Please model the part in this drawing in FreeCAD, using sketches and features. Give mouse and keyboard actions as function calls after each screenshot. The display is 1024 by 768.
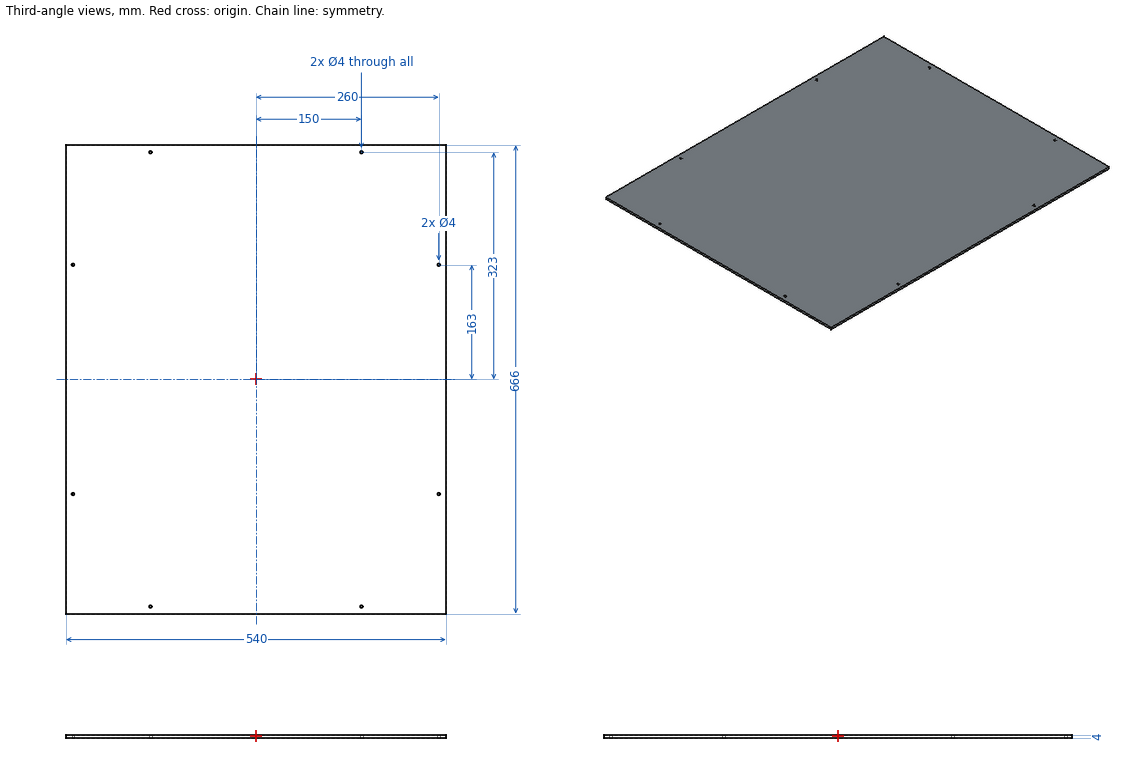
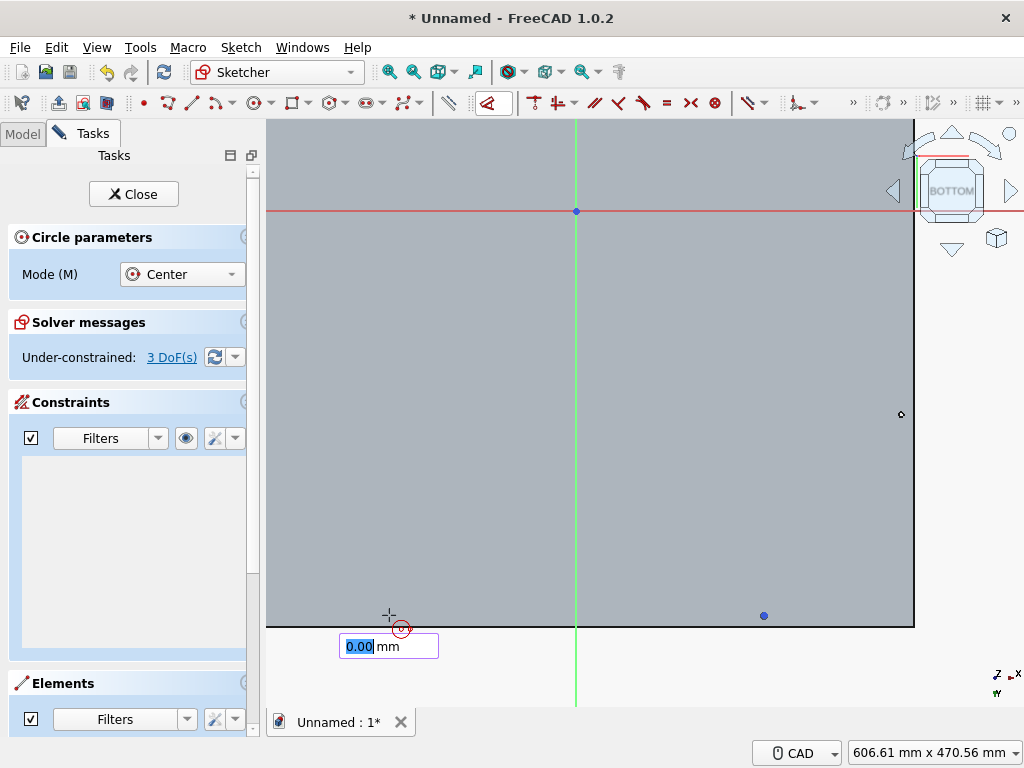
scroll(391, 613, up, 10)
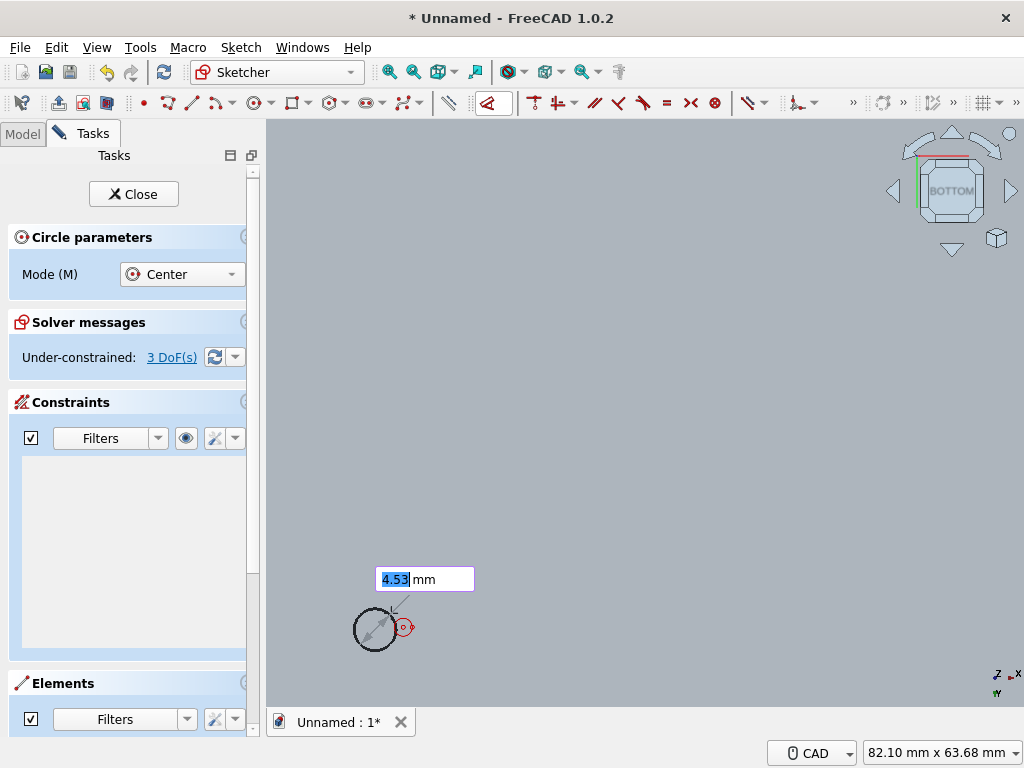
click(387, 606)
key(Escape)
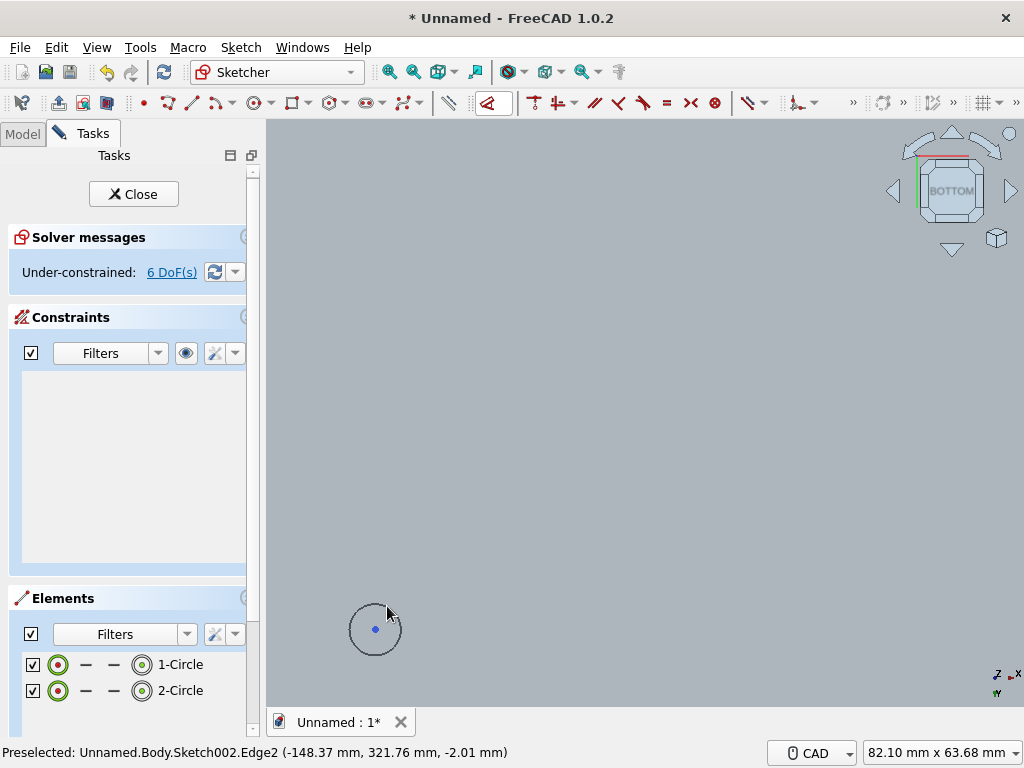
scroll(391, 613, down, 10)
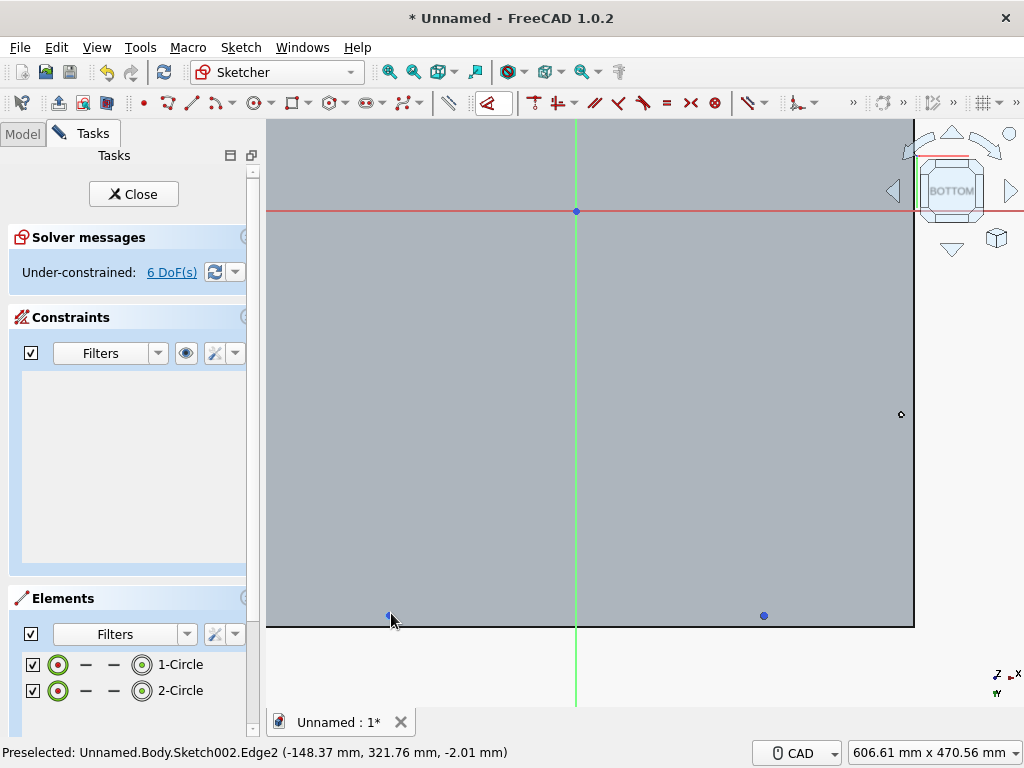
scroll(766, 614, up, 8)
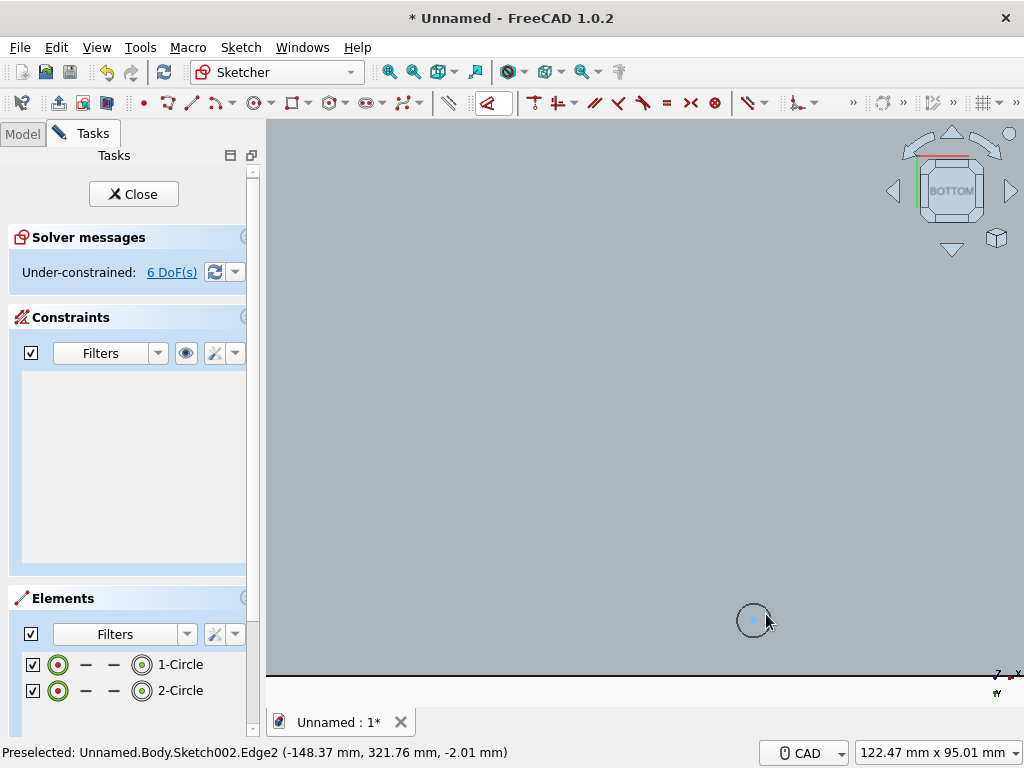
click(766, 609)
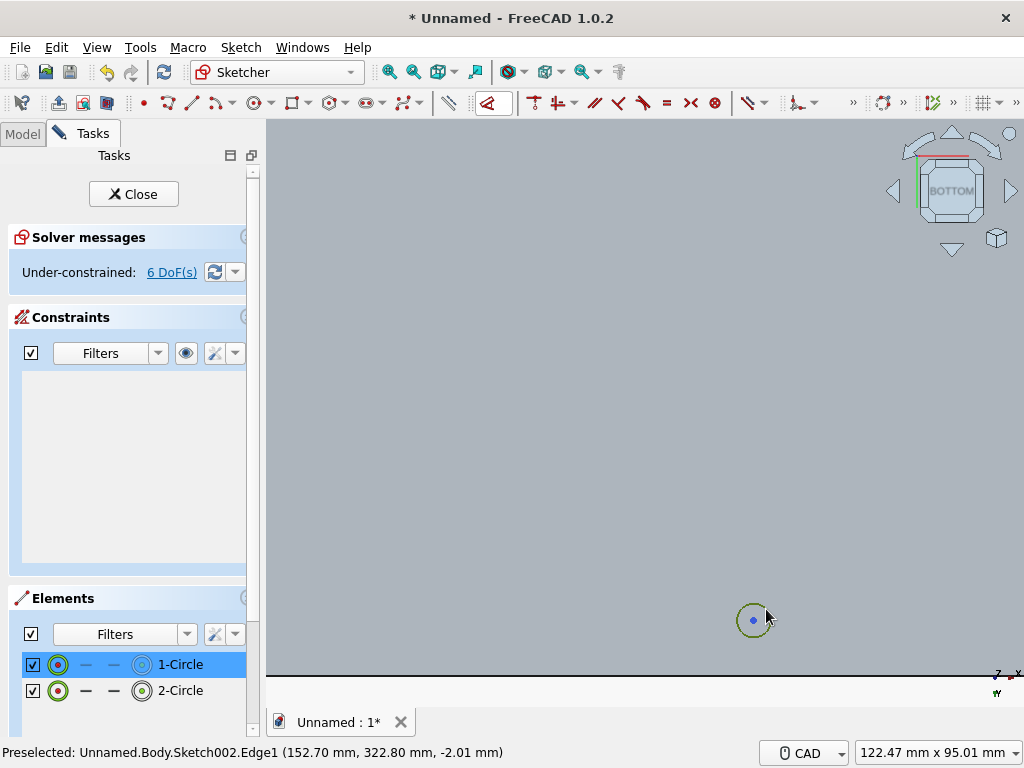
scroll(767, 614, down, 8)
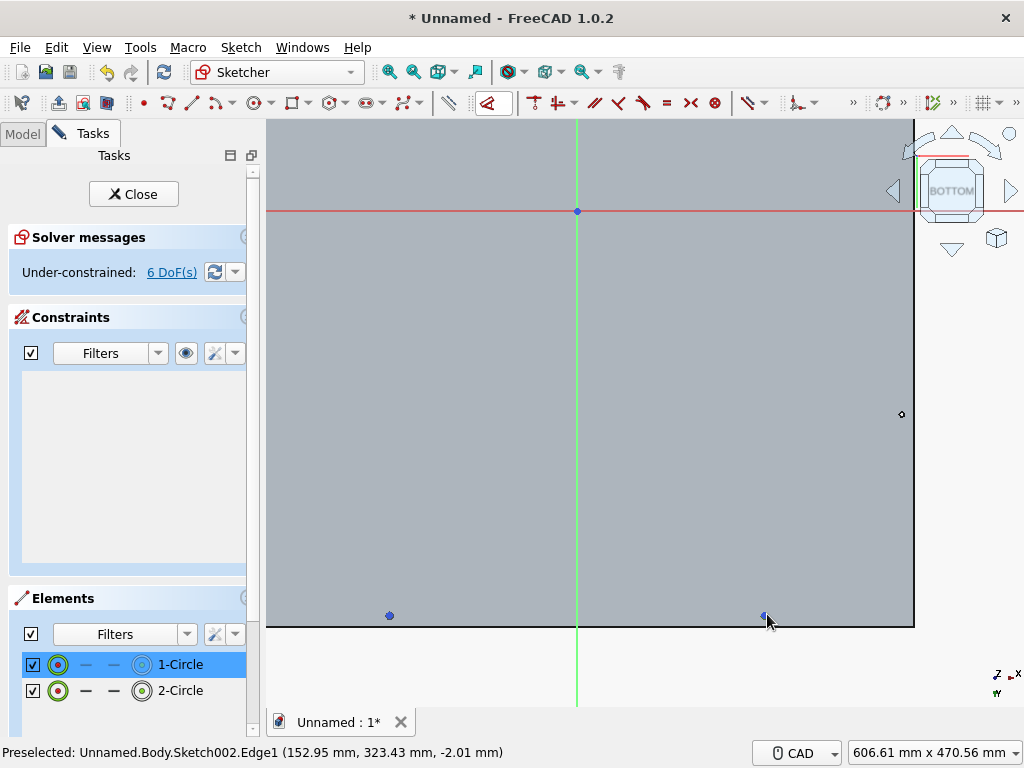
scroll(392, 614, up, 7)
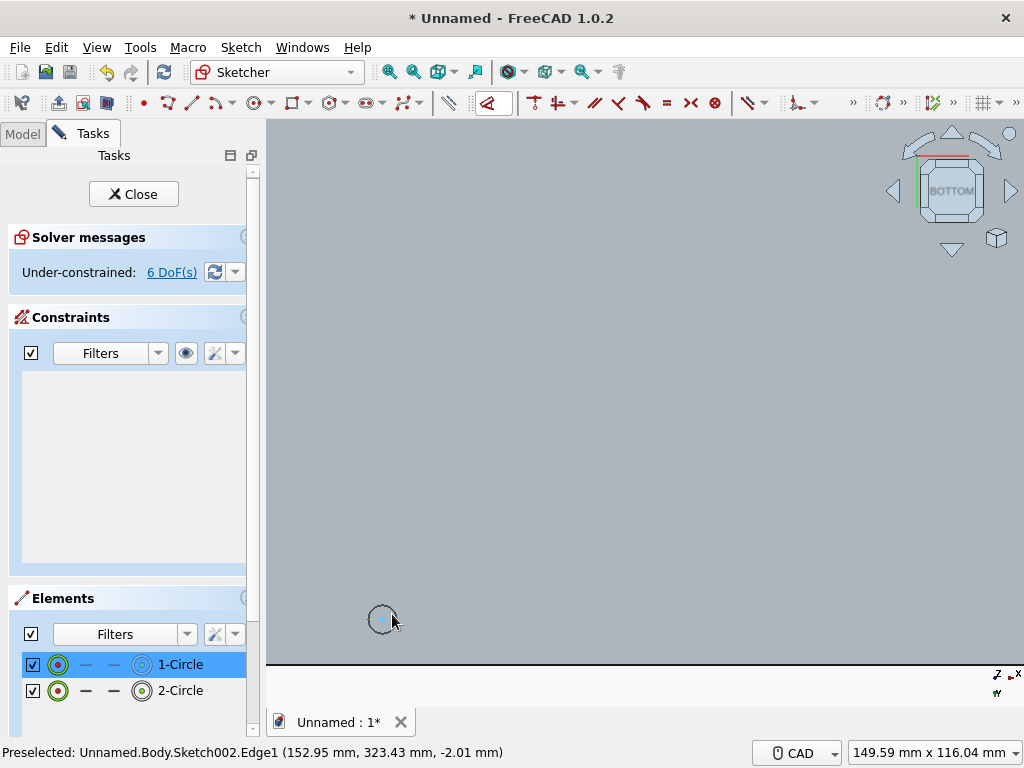
click(393, 610)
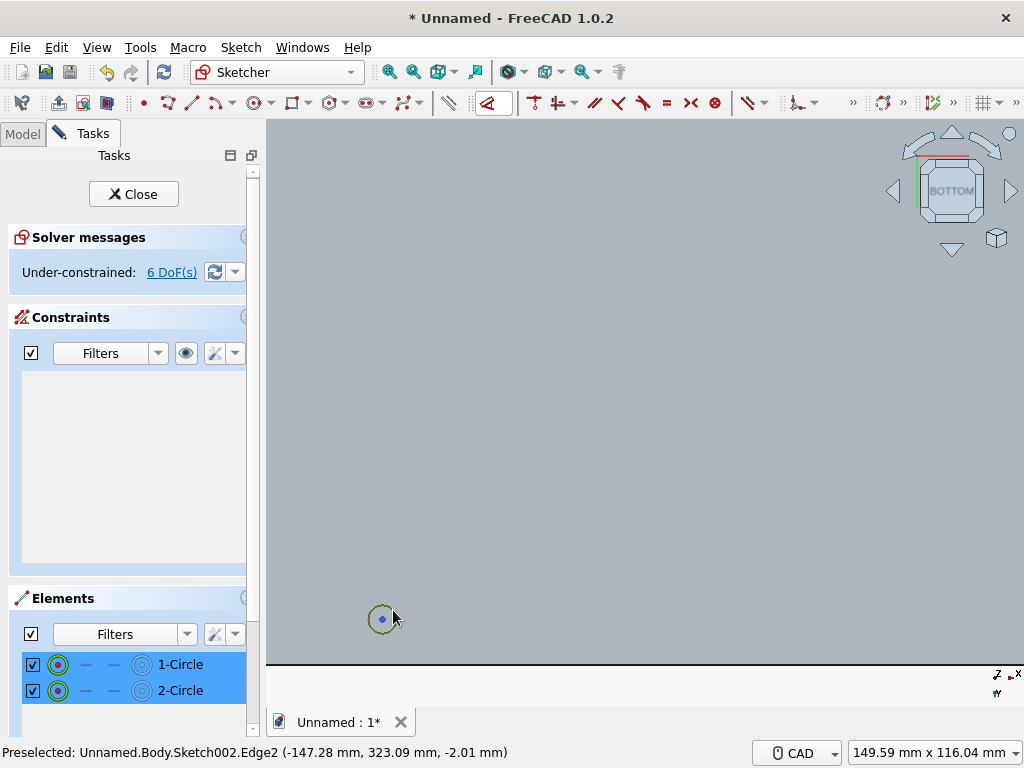
key(e)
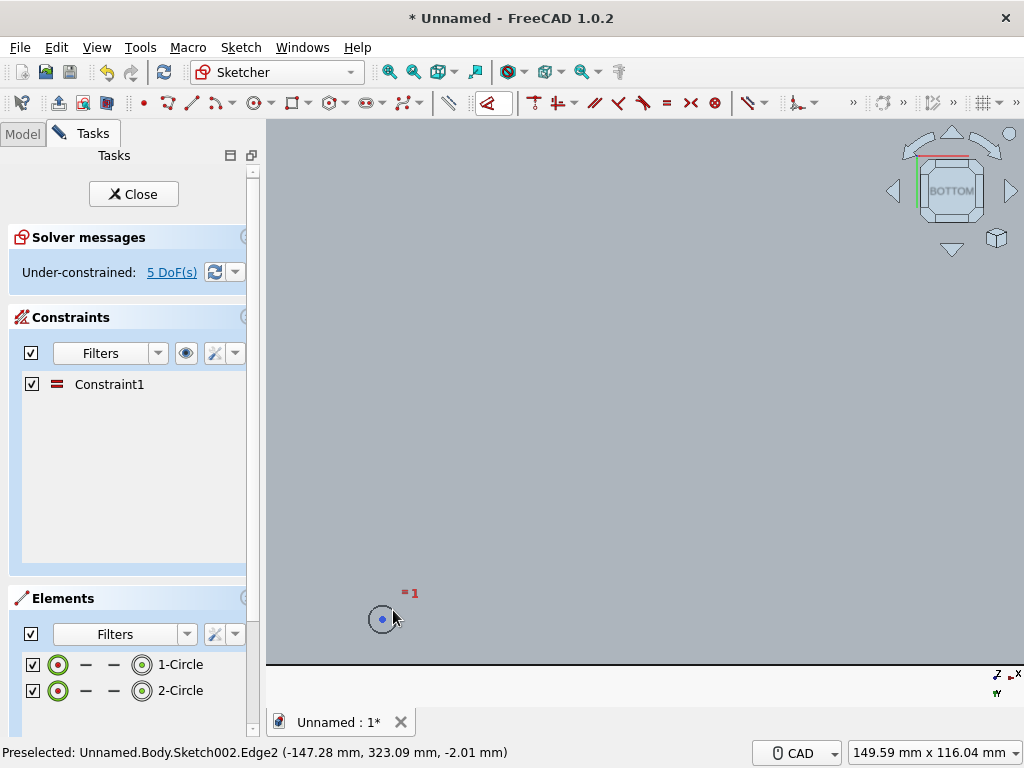
scroll(391, 613, down, 7)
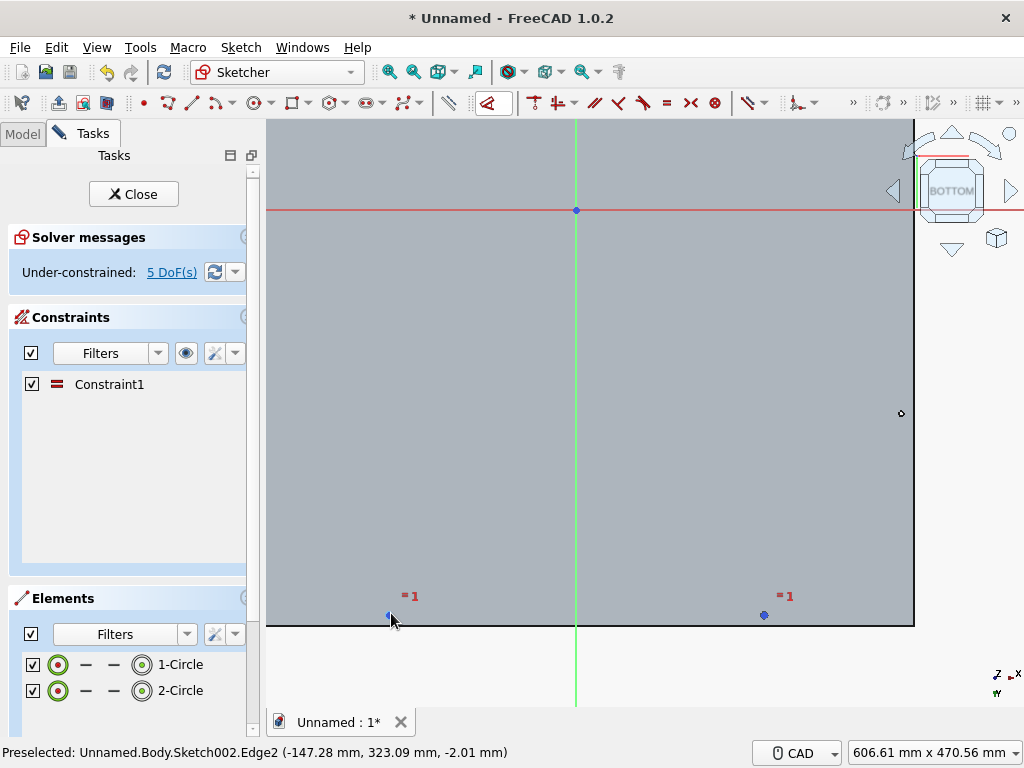
click(764, 615)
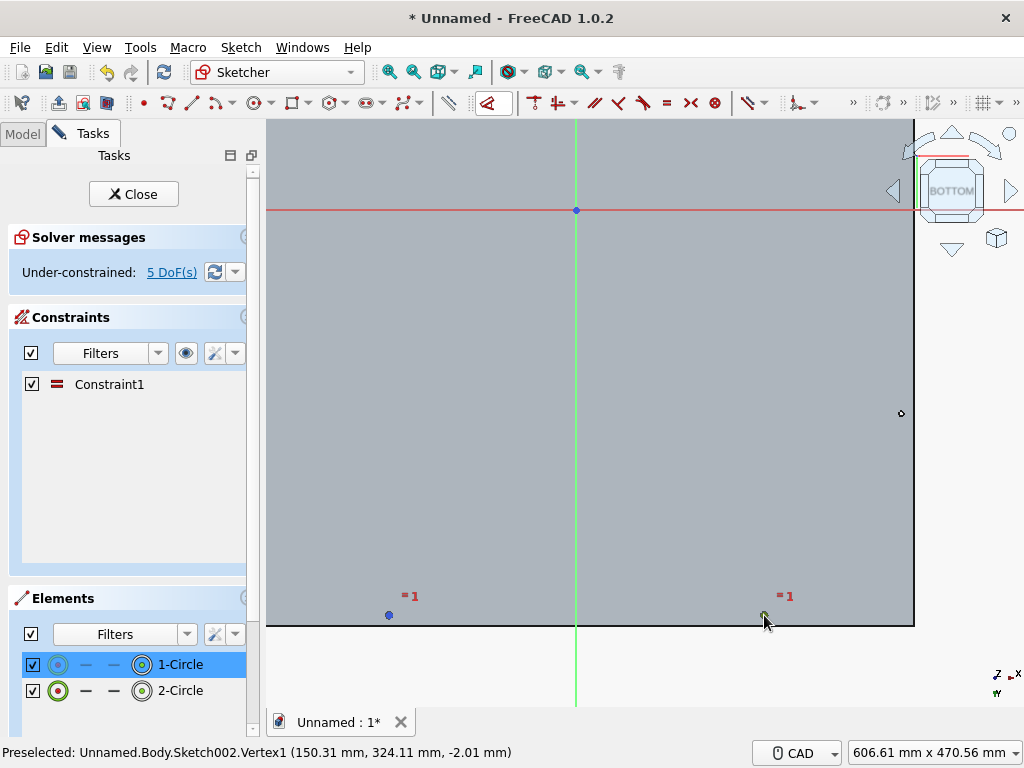
click(389, 615)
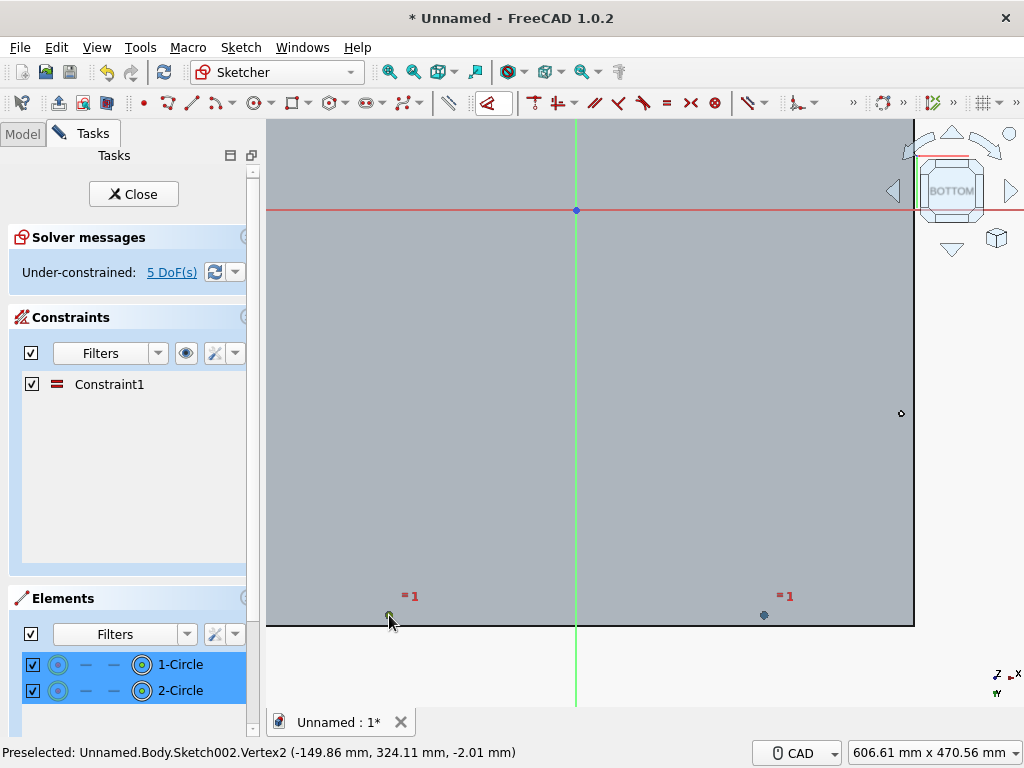
click(576, 641)